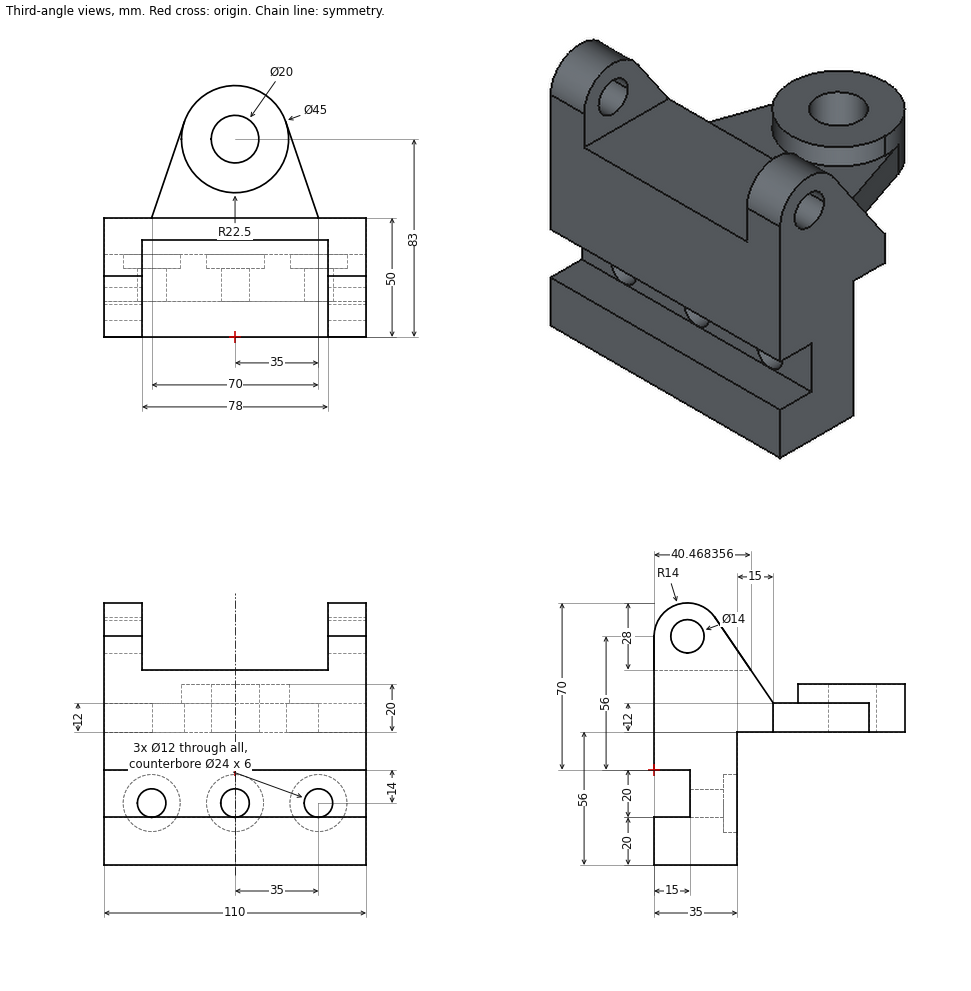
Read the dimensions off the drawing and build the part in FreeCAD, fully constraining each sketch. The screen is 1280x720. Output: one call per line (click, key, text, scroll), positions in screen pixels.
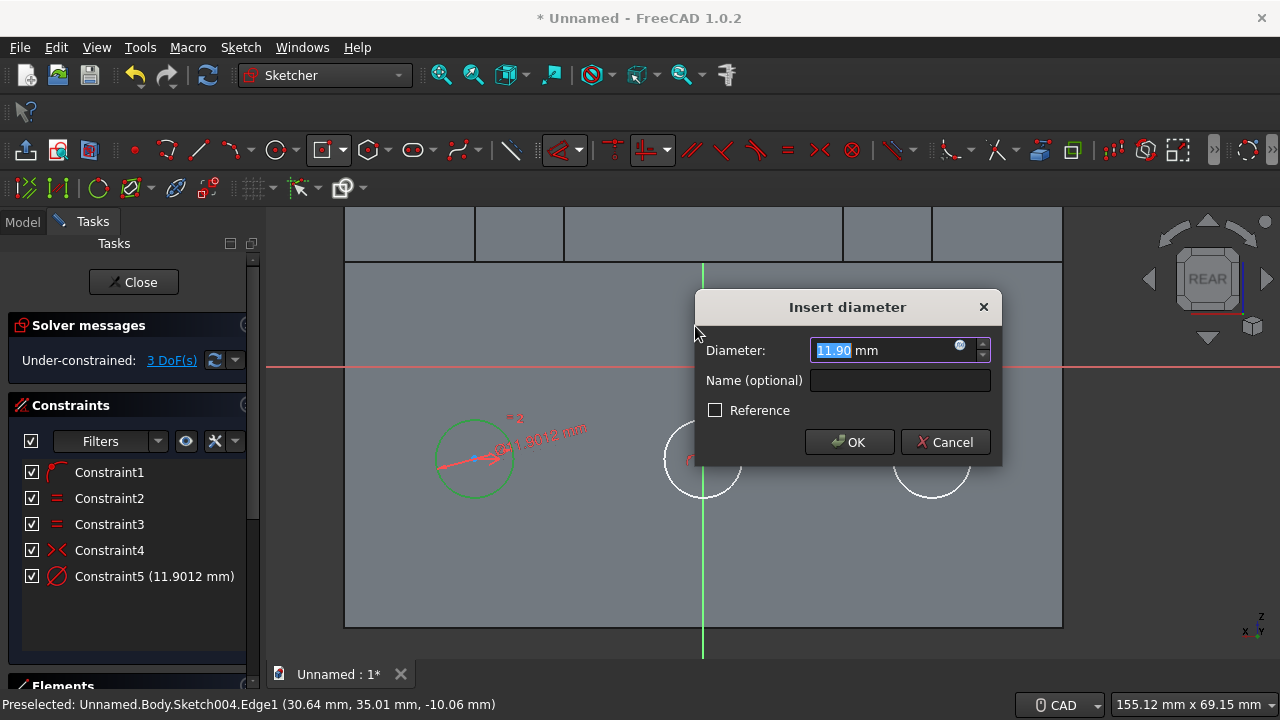
text(12)
key(Return)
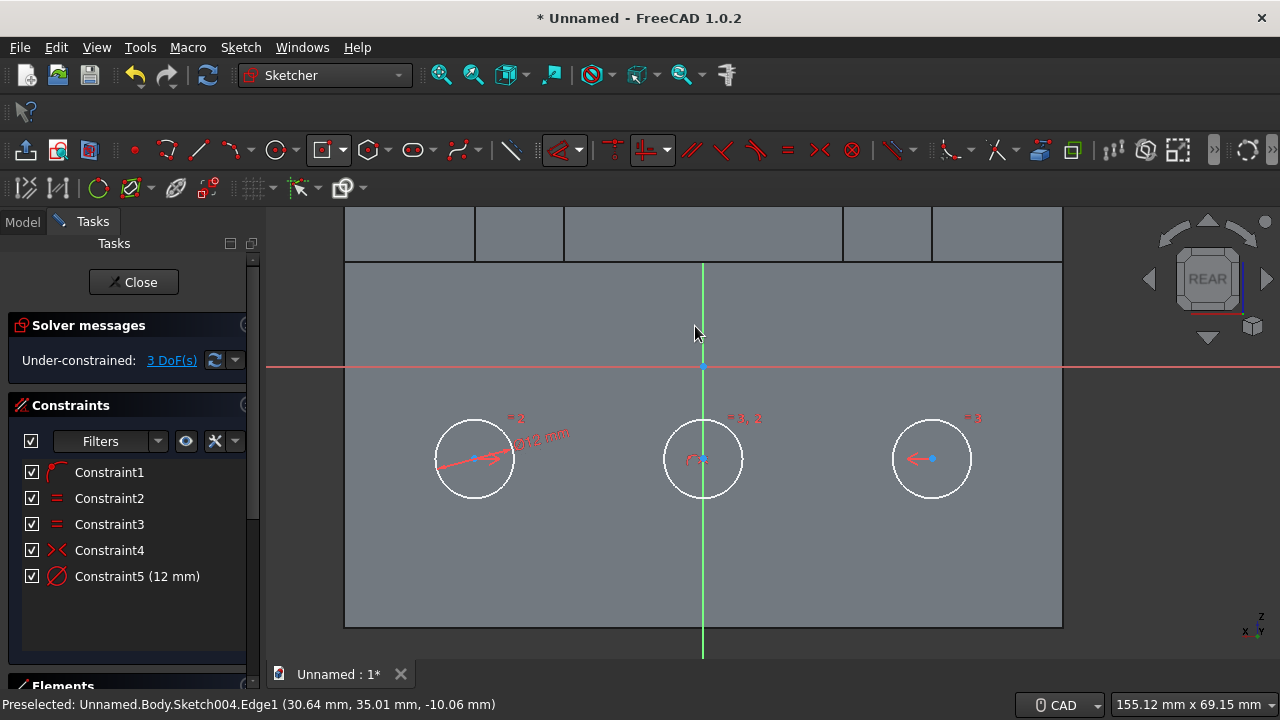
click(475, 459)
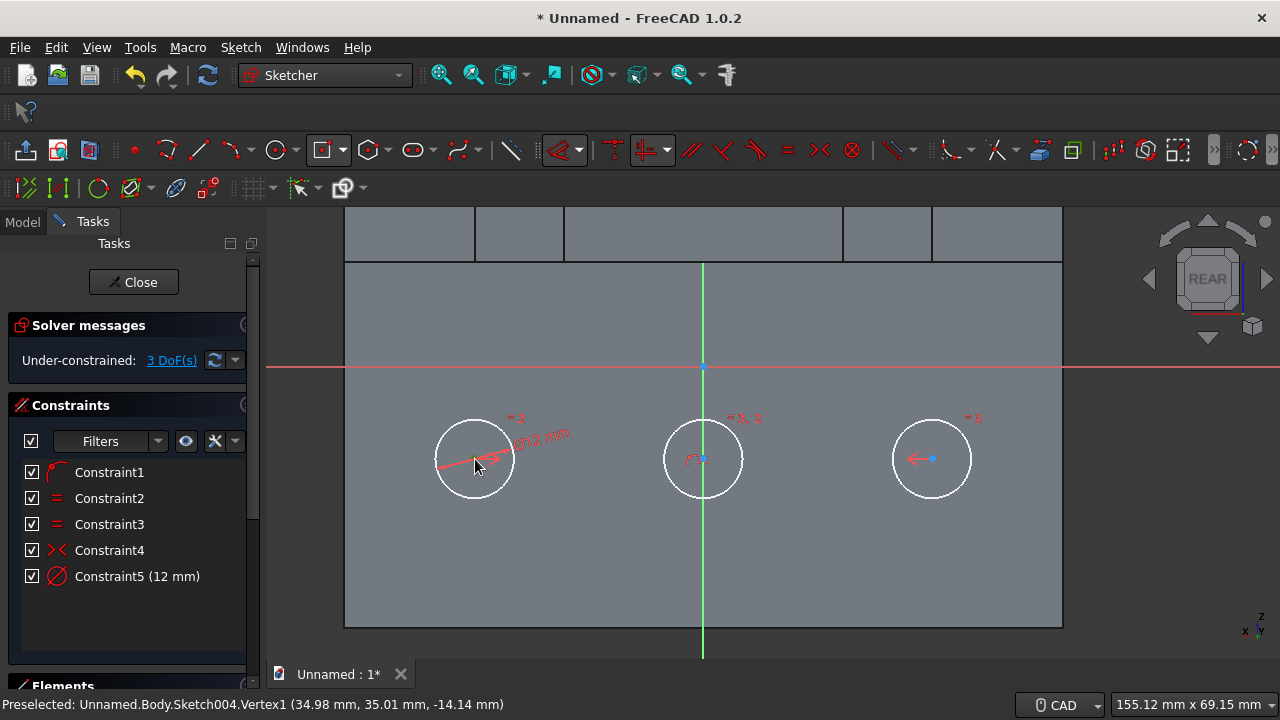
click(582, 150)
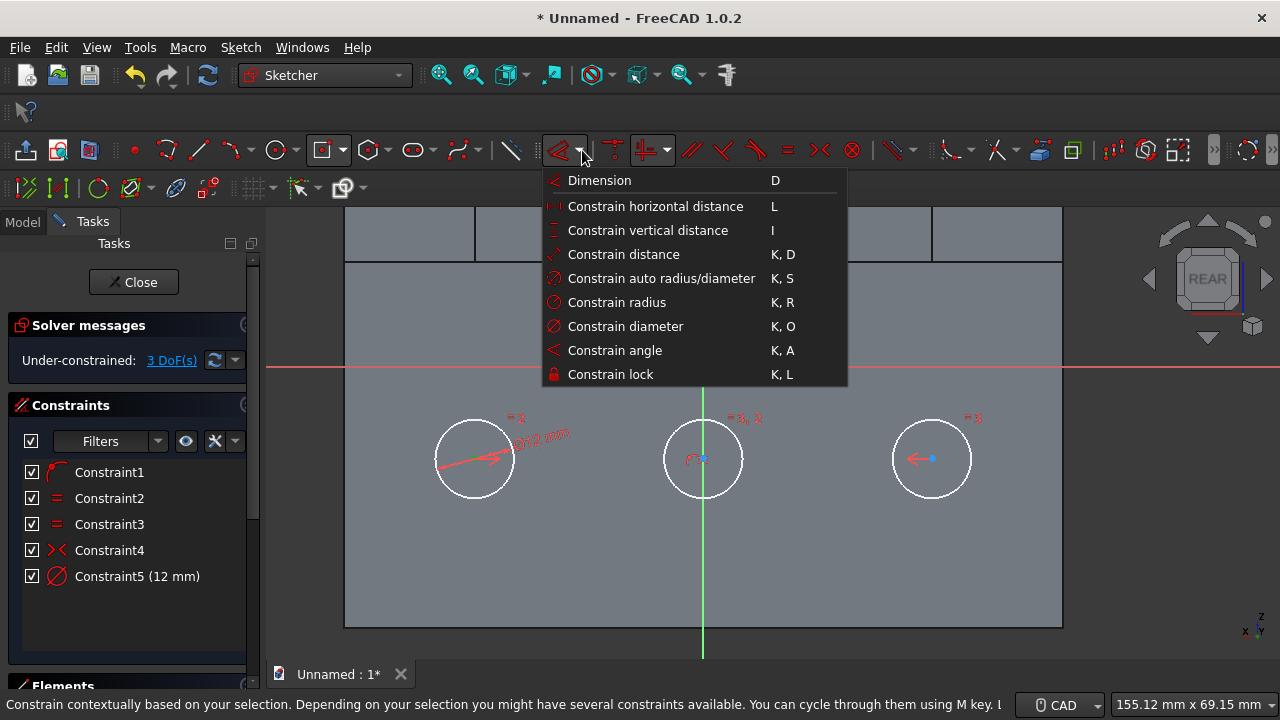
click(695, 206)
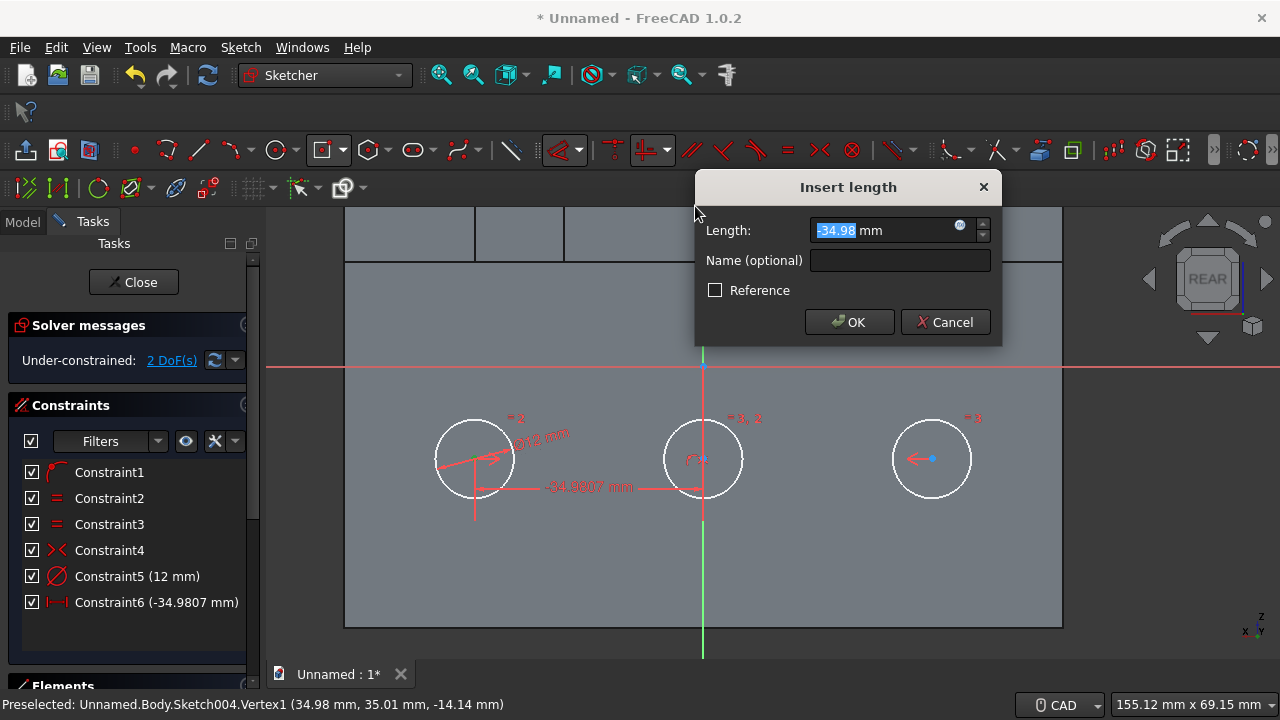
text(-35)
key(Return)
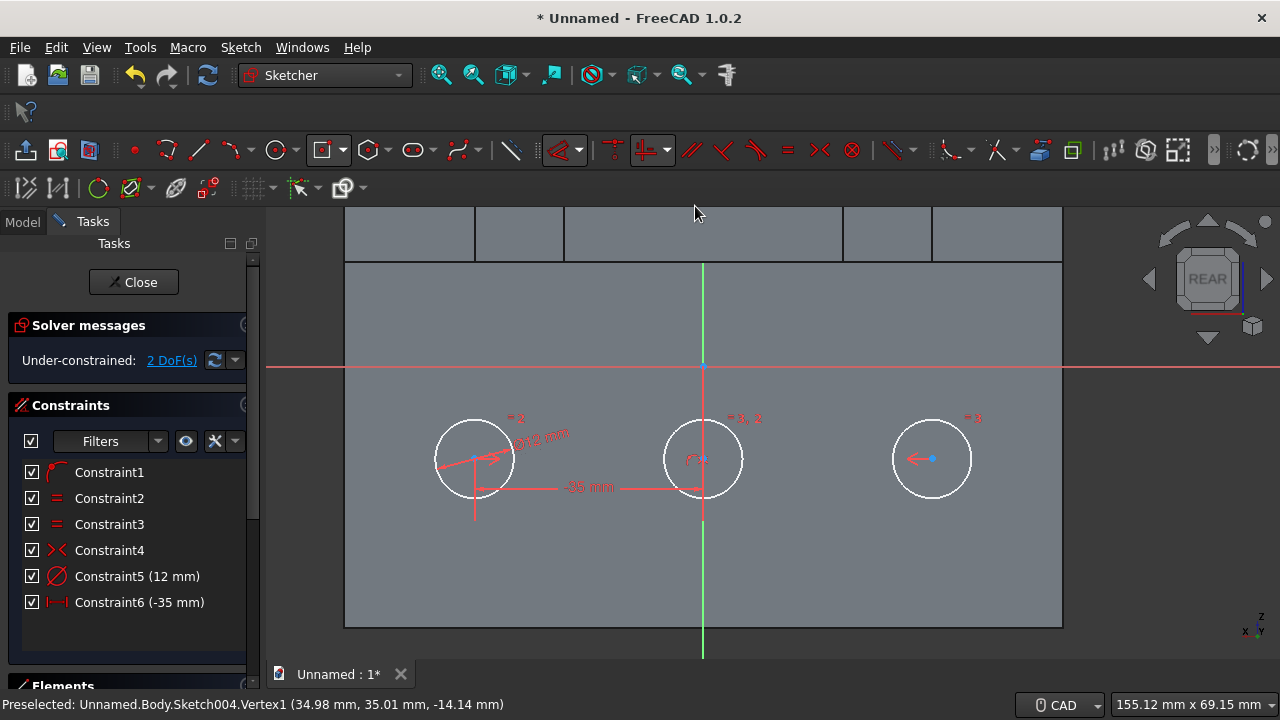
click(475, 459)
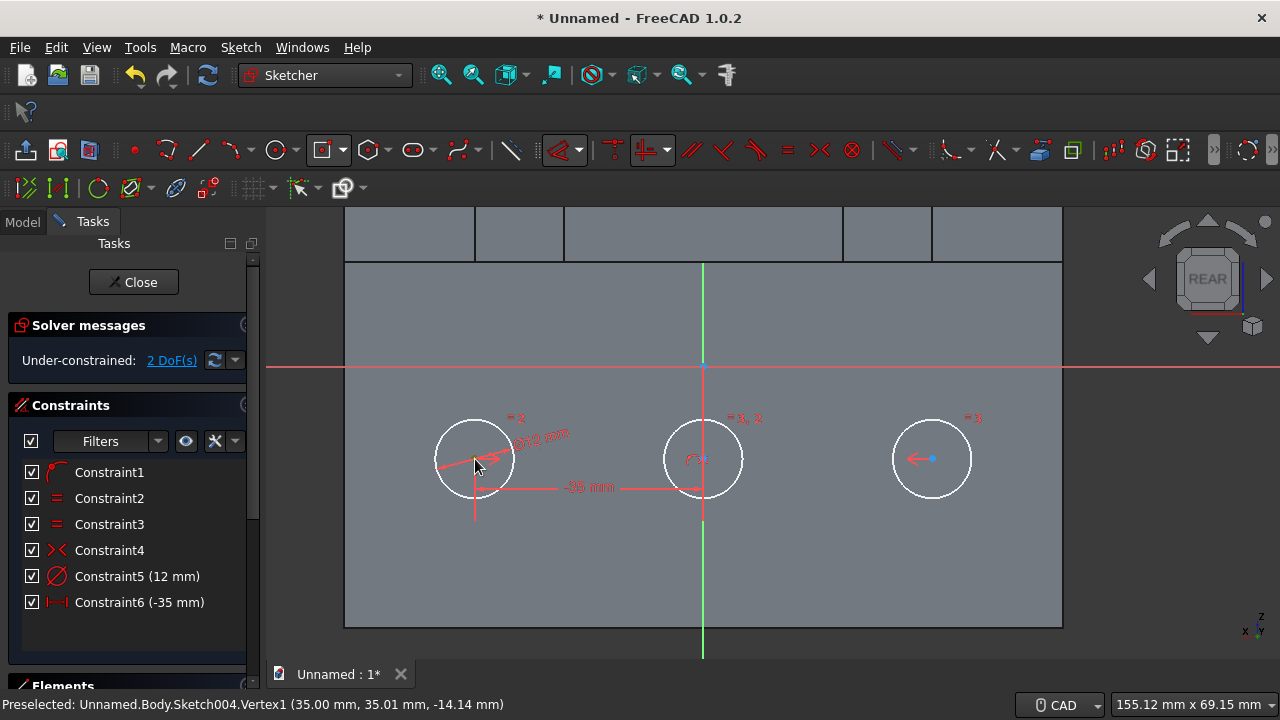
key(i)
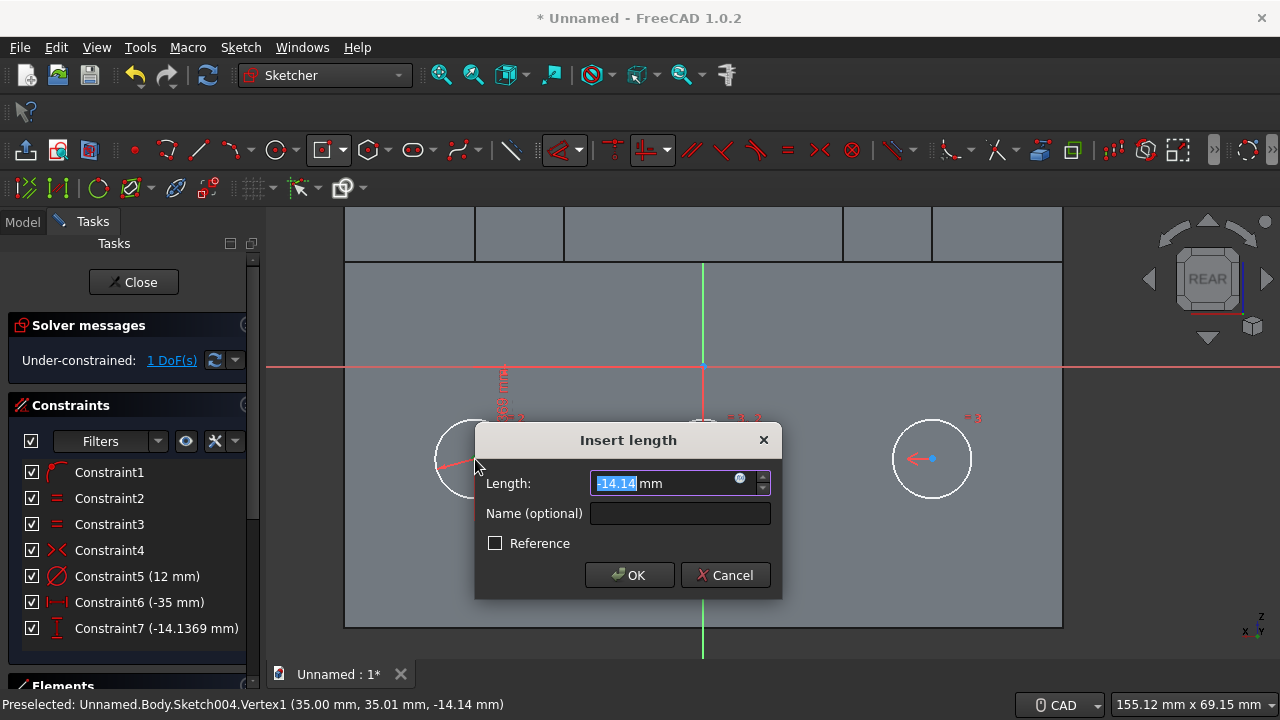
text(-14)
key(Return)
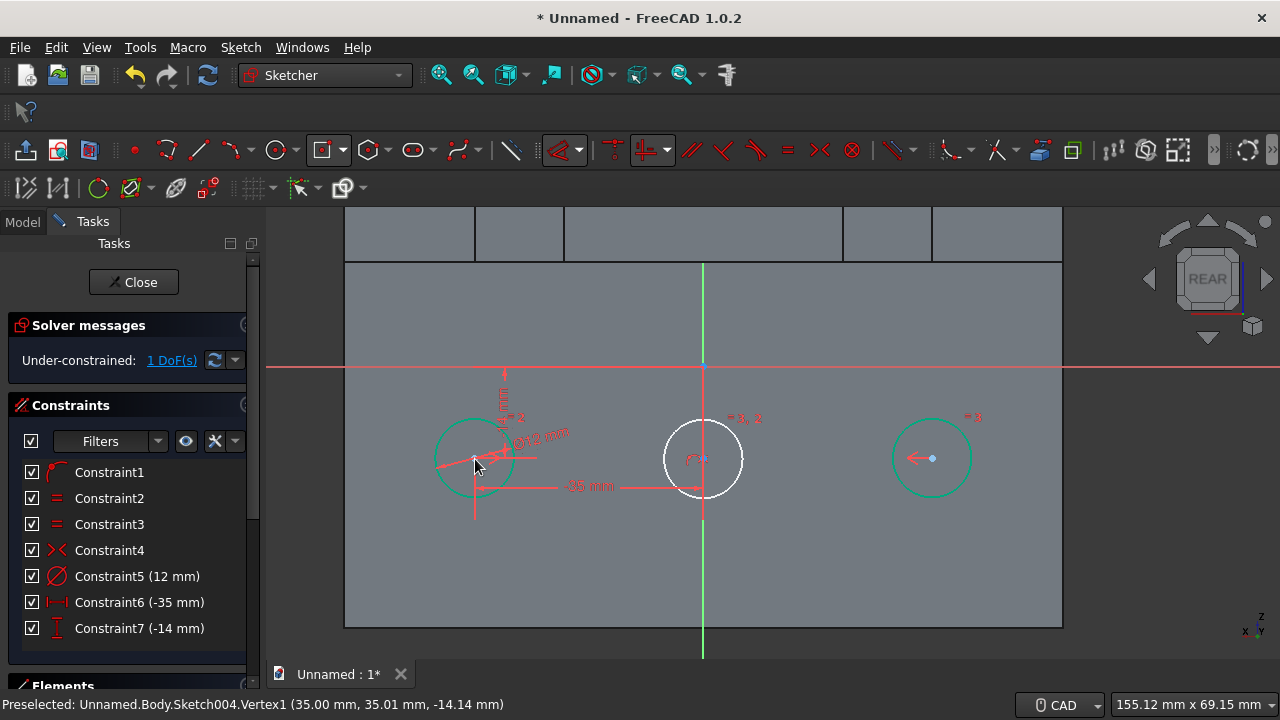
click(703, 459)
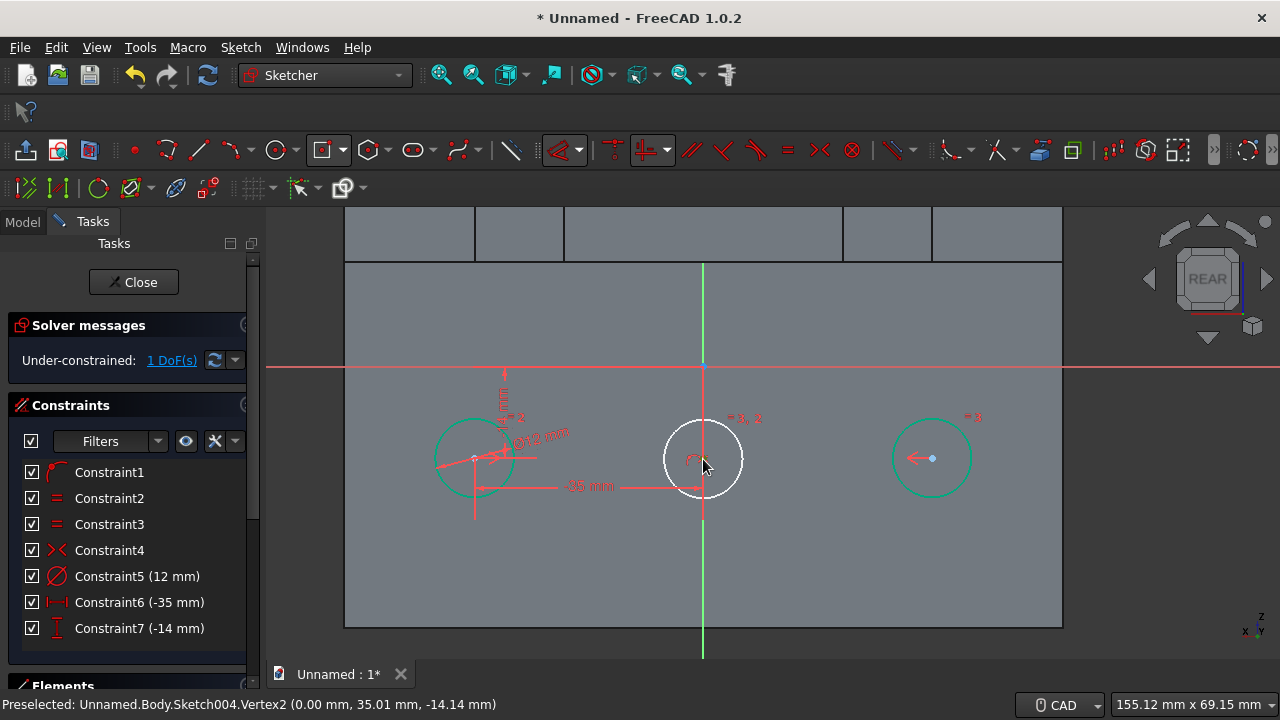
key(i)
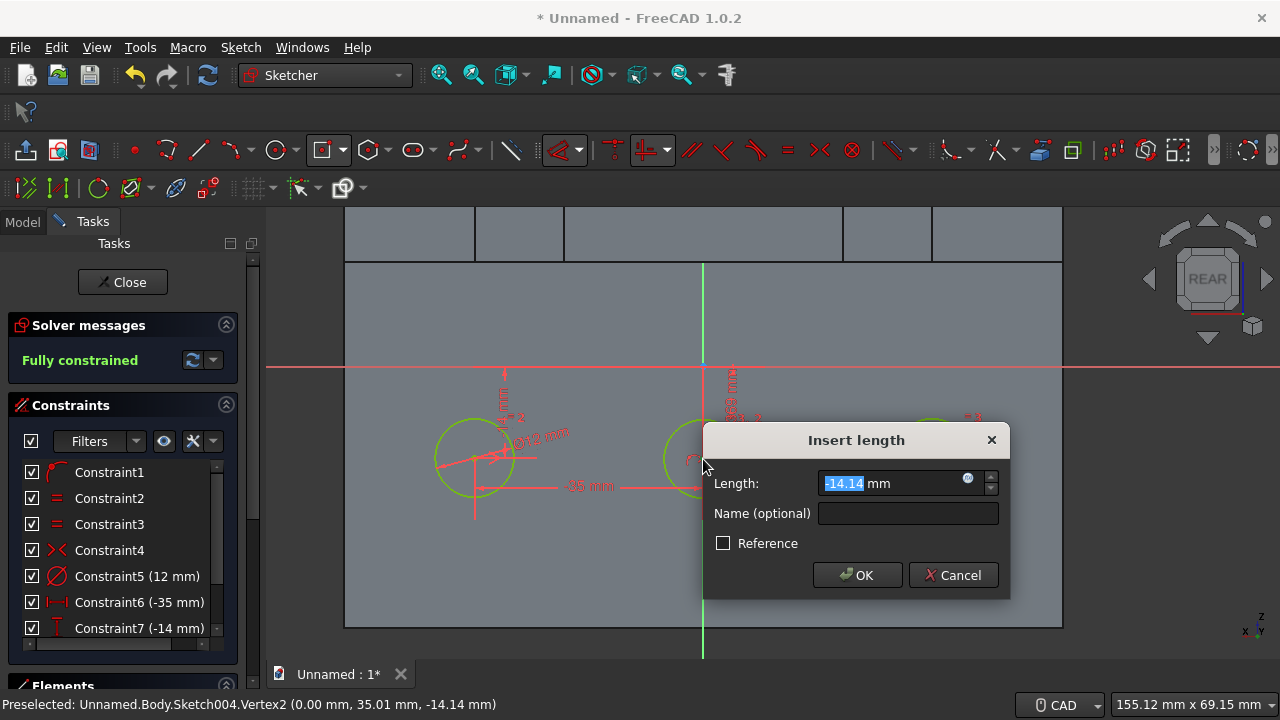
text(-14)
key(Return)